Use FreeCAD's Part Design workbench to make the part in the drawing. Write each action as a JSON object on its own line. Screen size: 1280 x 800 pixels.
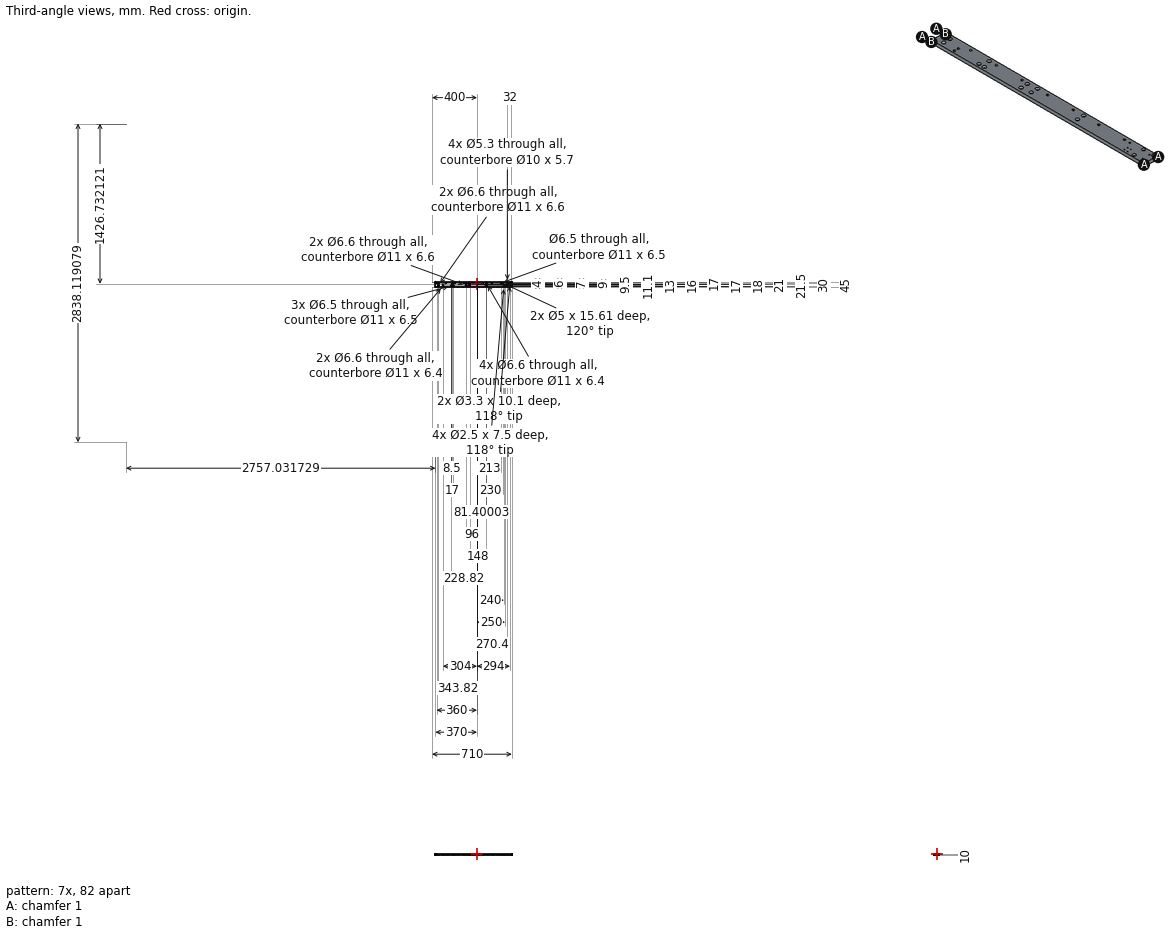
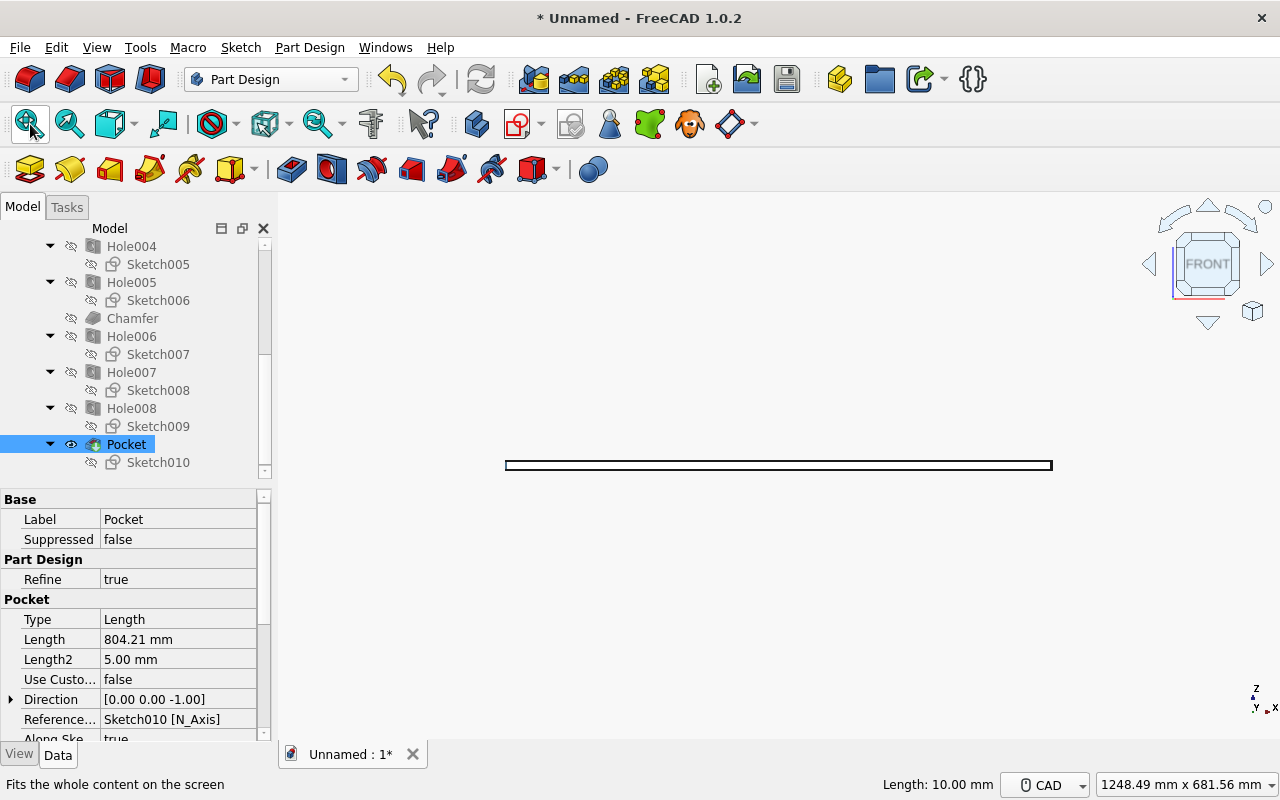
{"action": "key", "text": "3"}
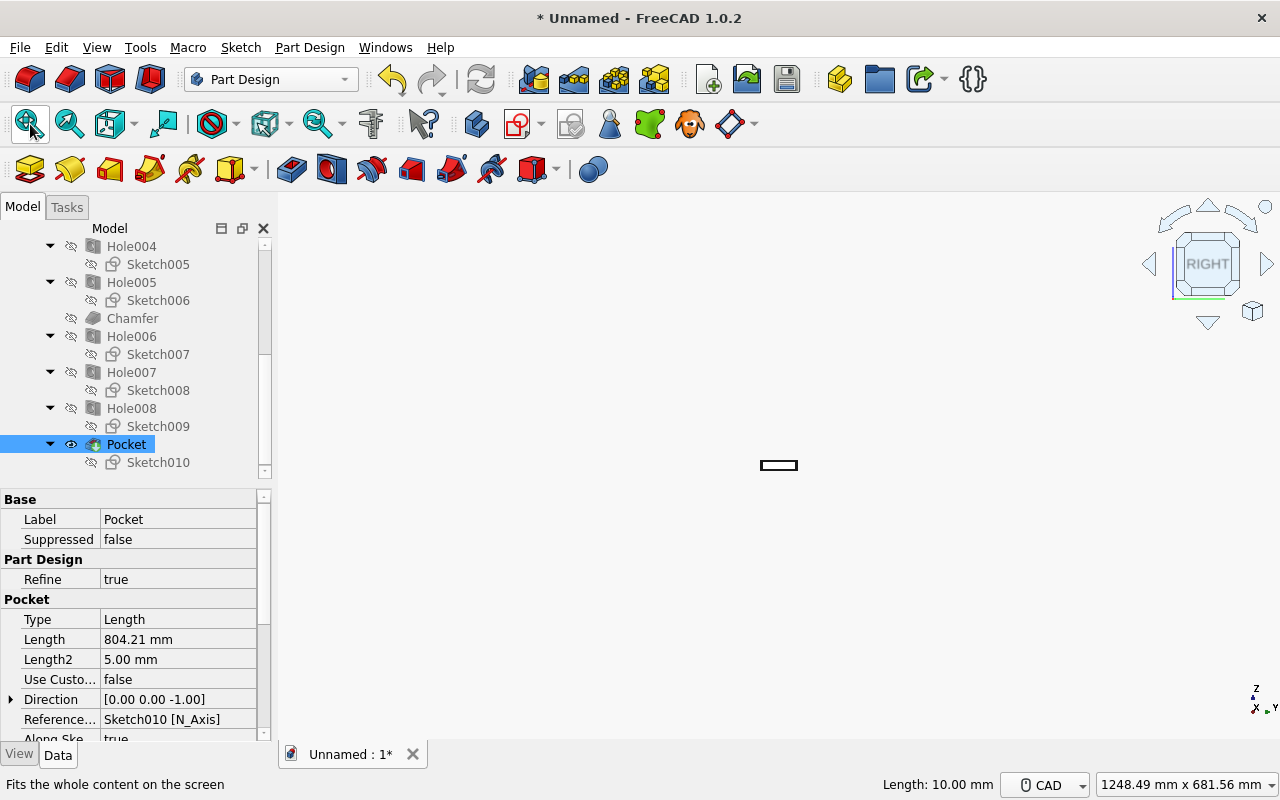
{"action": "left_click", "coordinate": [30, 124]}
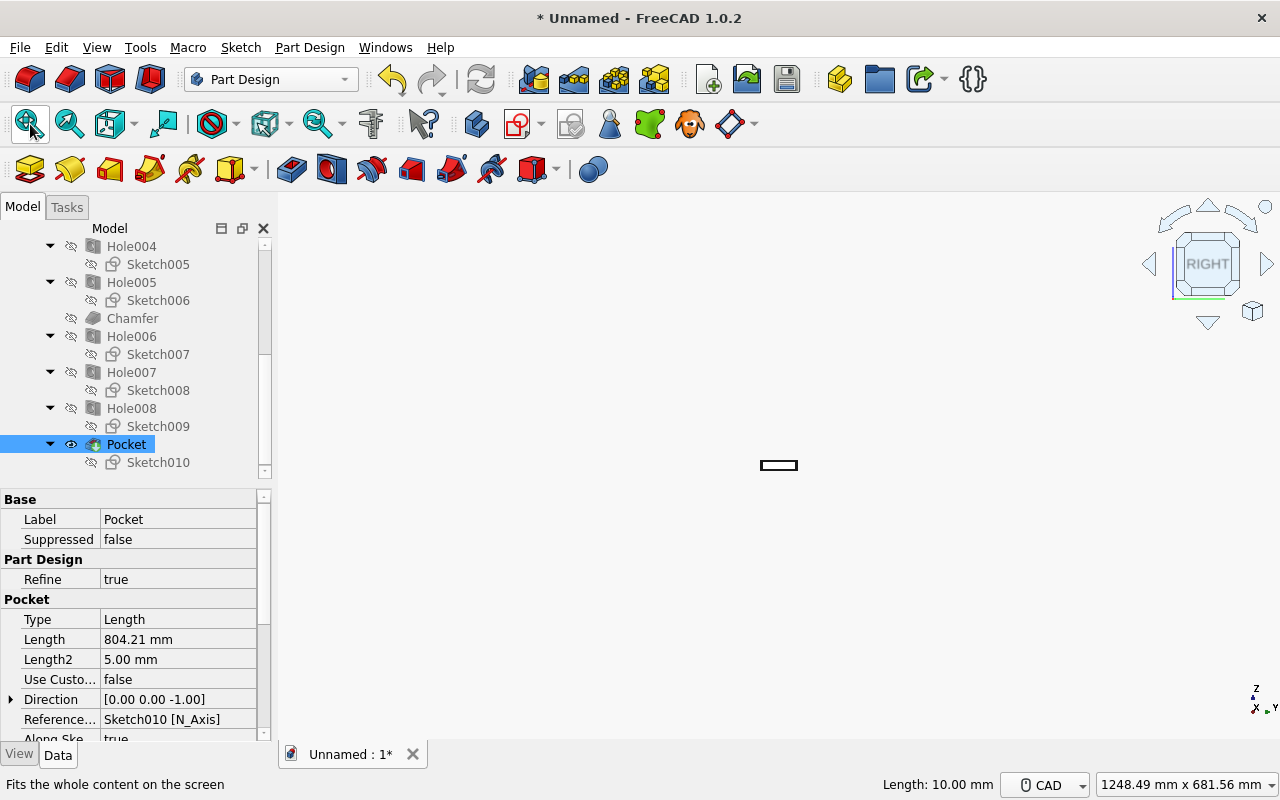
{"action": "scroll", "coordinate": [797, 464], "scroll_direction": "up", "scroll_amount": 9}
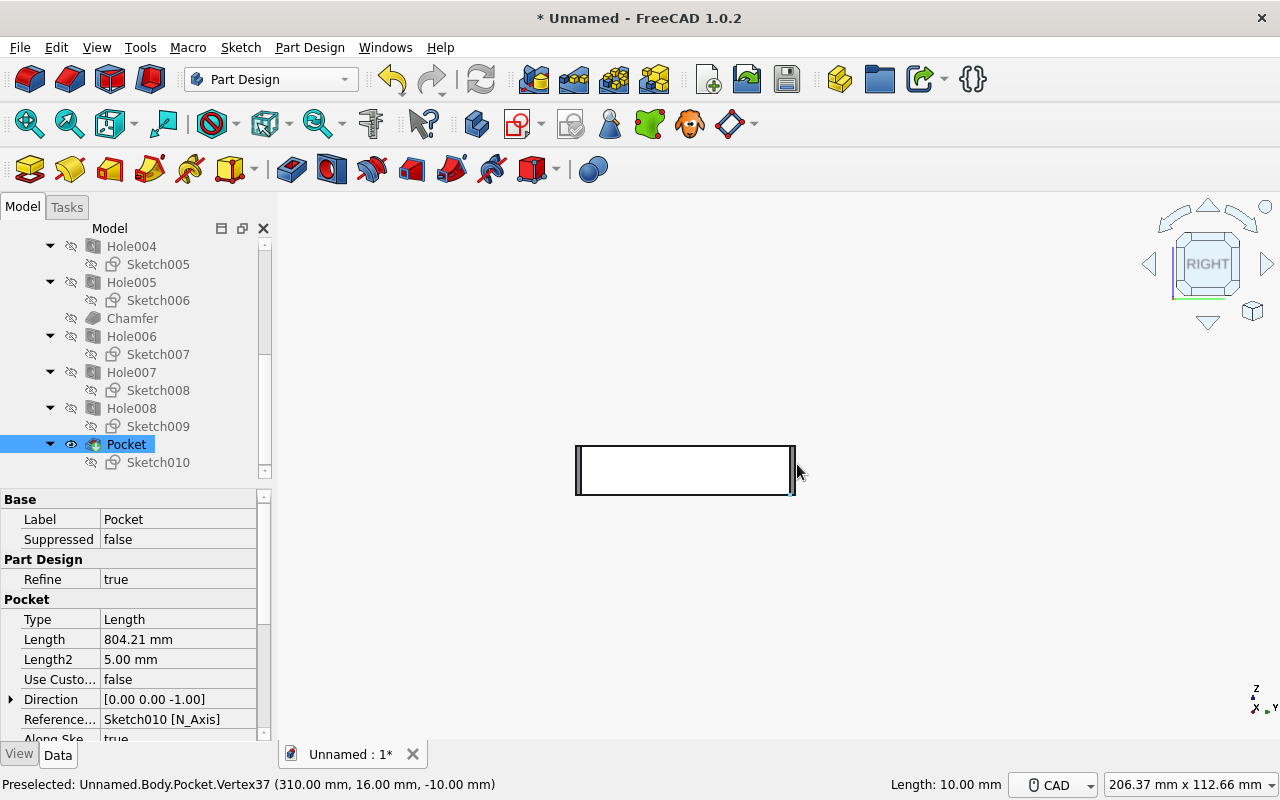
{"action": "left_click", "coordinate": [30, 124]}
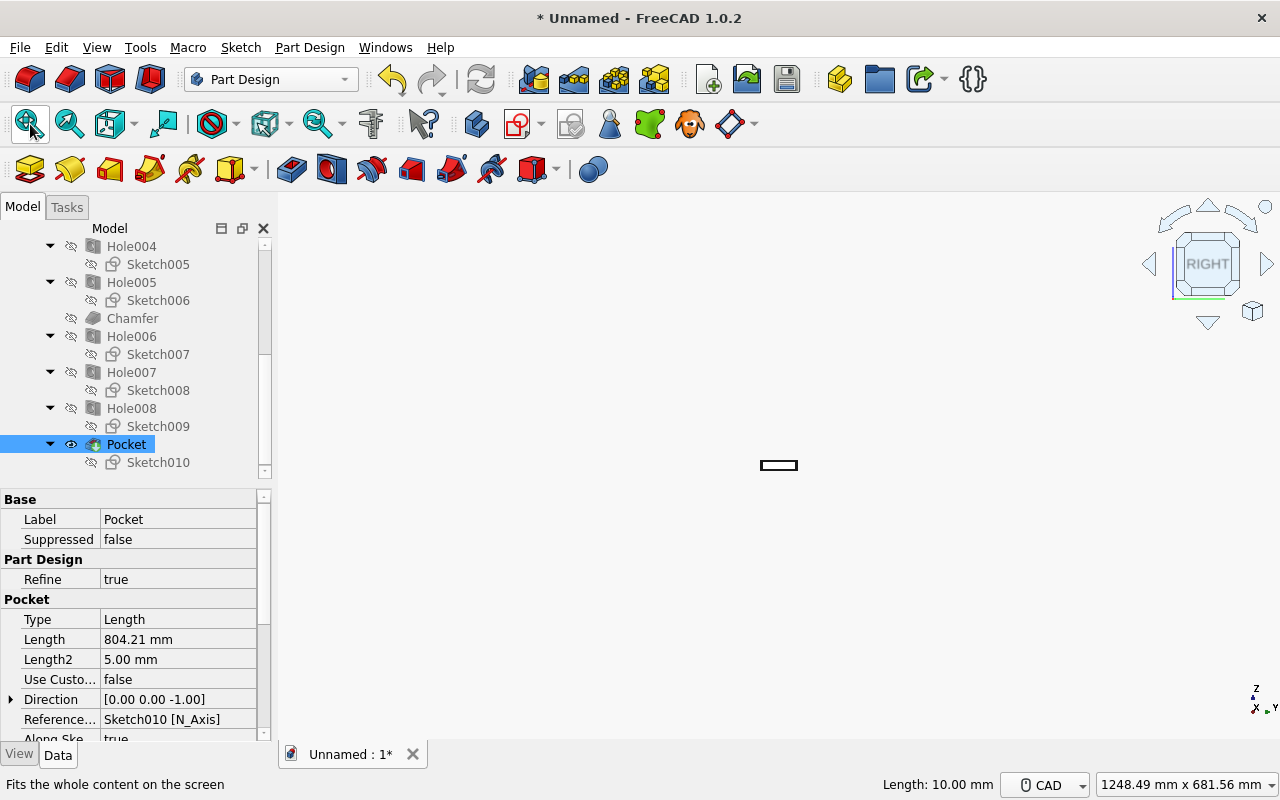
{"action": "key", "text": "5"}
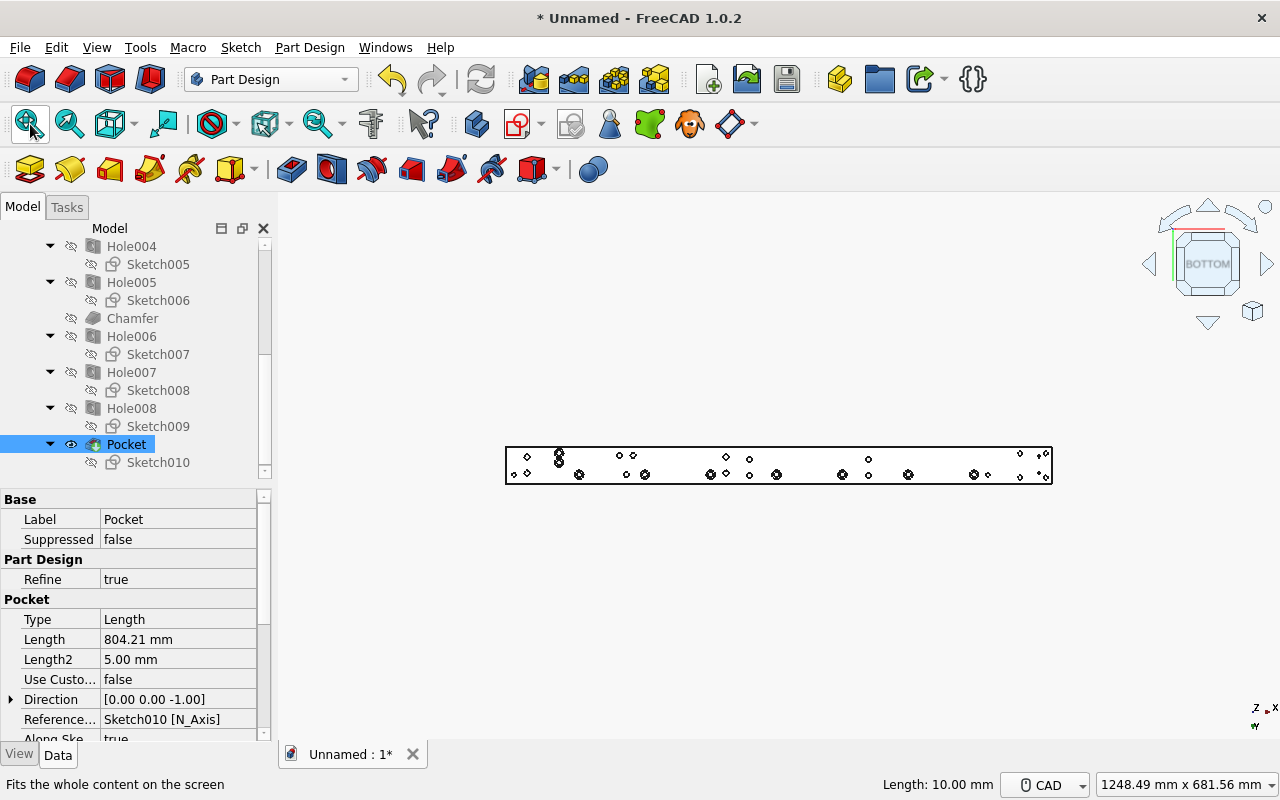
{"action": "scroll", "coordinate": [506, 483], "scroll_direction": "up", "scroll_amount": 9}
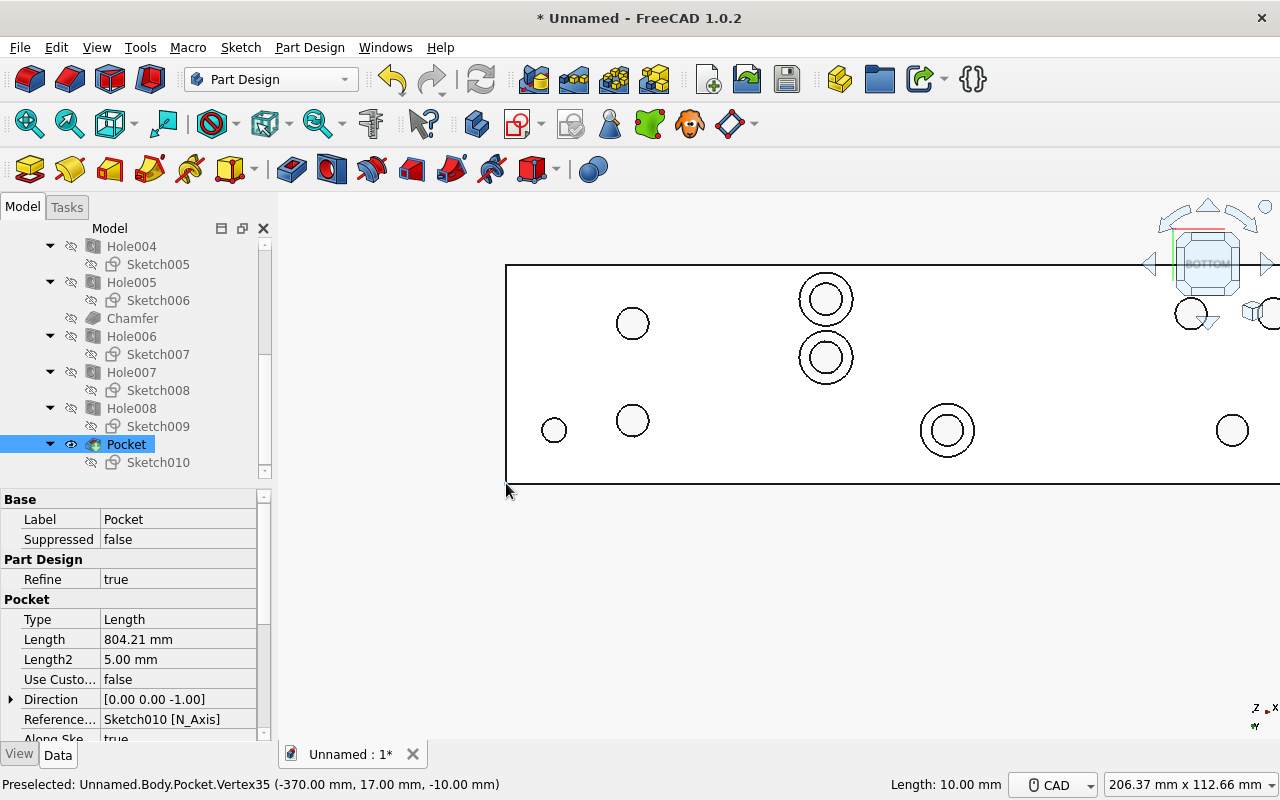
{"action": "left_click", "coordinate": [30, 124]}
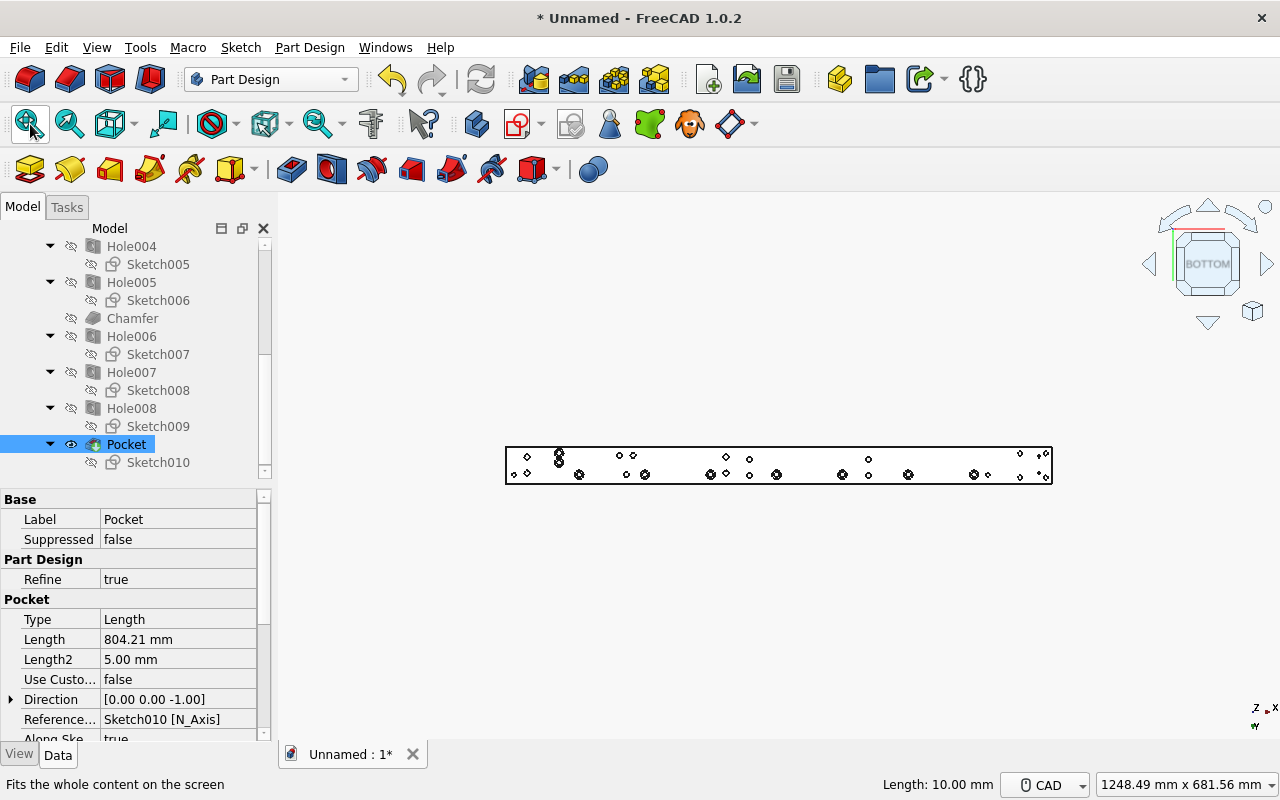
{"action": "key", "text": "4"}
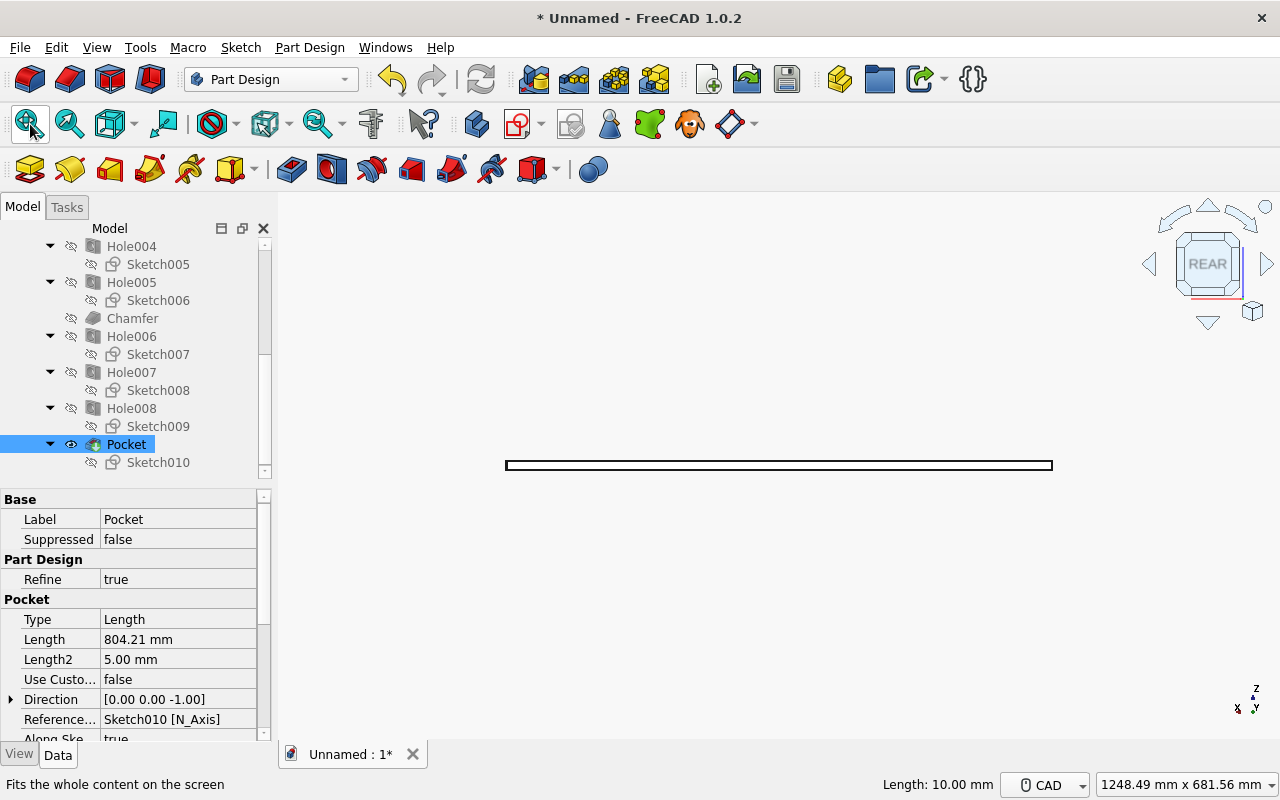
{"action": "scroll", "coordinate": [1052, 464], "scroll_direction": "up", "scroll_amount": 9}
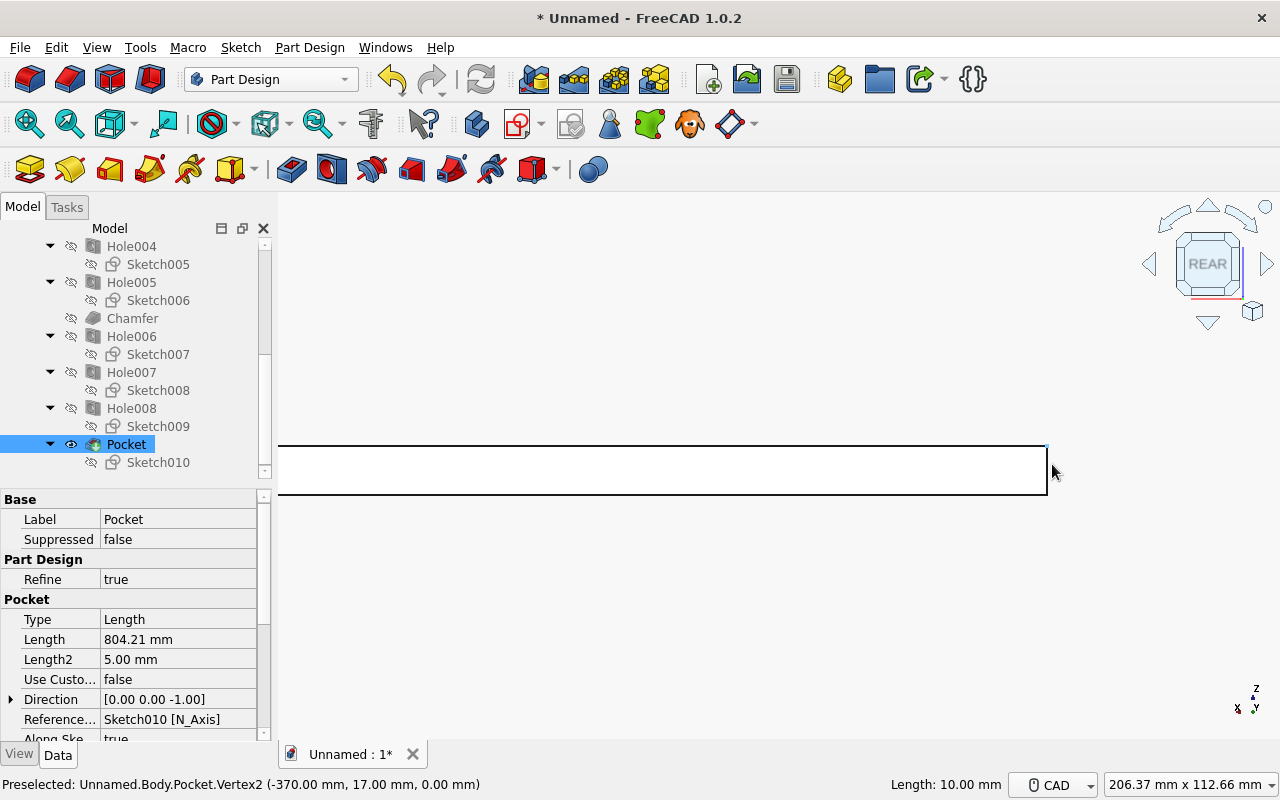
{"action": "left_click", "coordinate": [1047, 470], "text": "ctrl"}